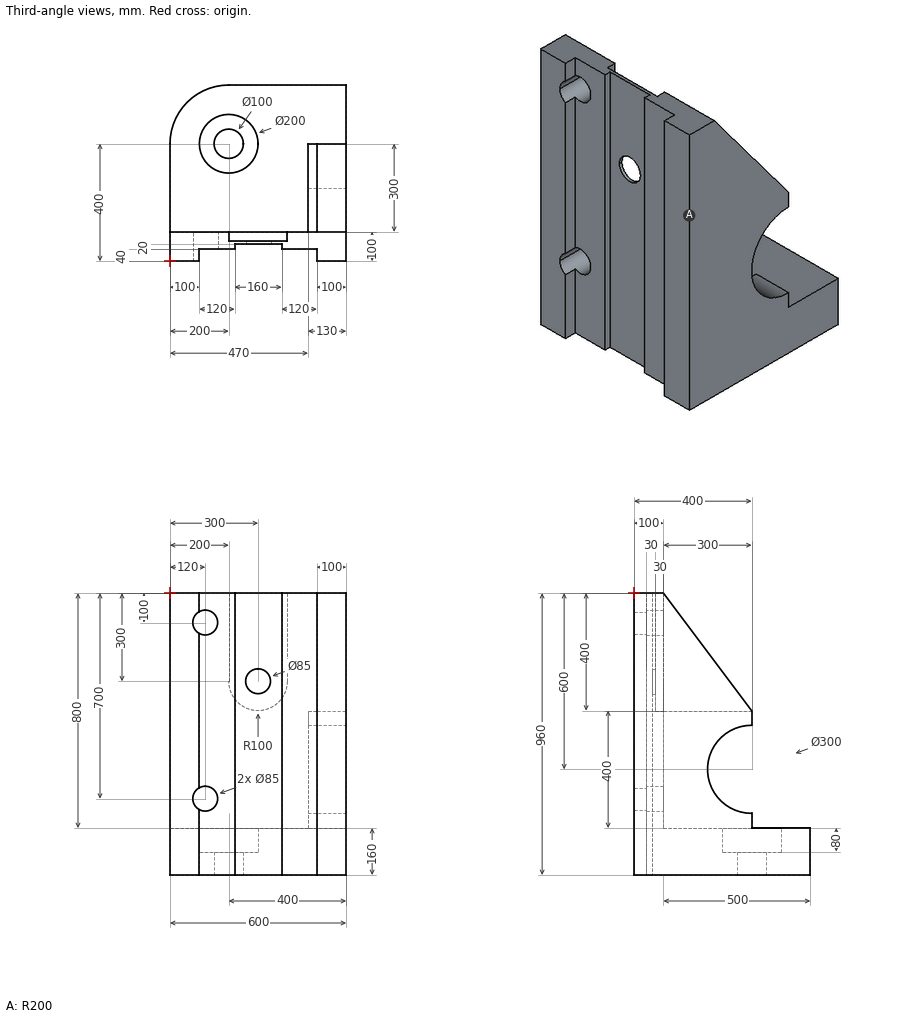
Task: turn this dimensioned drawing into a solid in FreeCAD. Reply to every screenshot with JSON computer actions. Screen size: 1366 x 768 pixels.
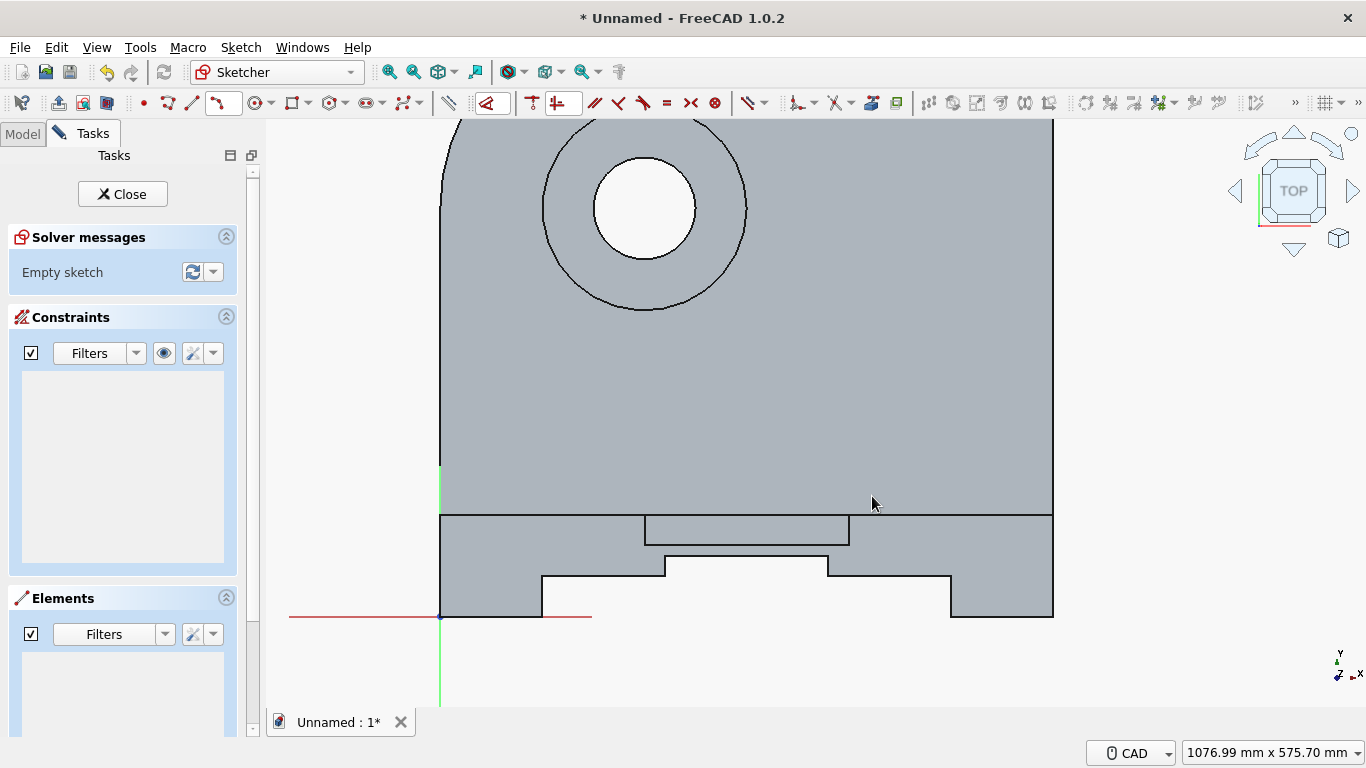
{"action": "left_click", "coordinate": [292, 104]}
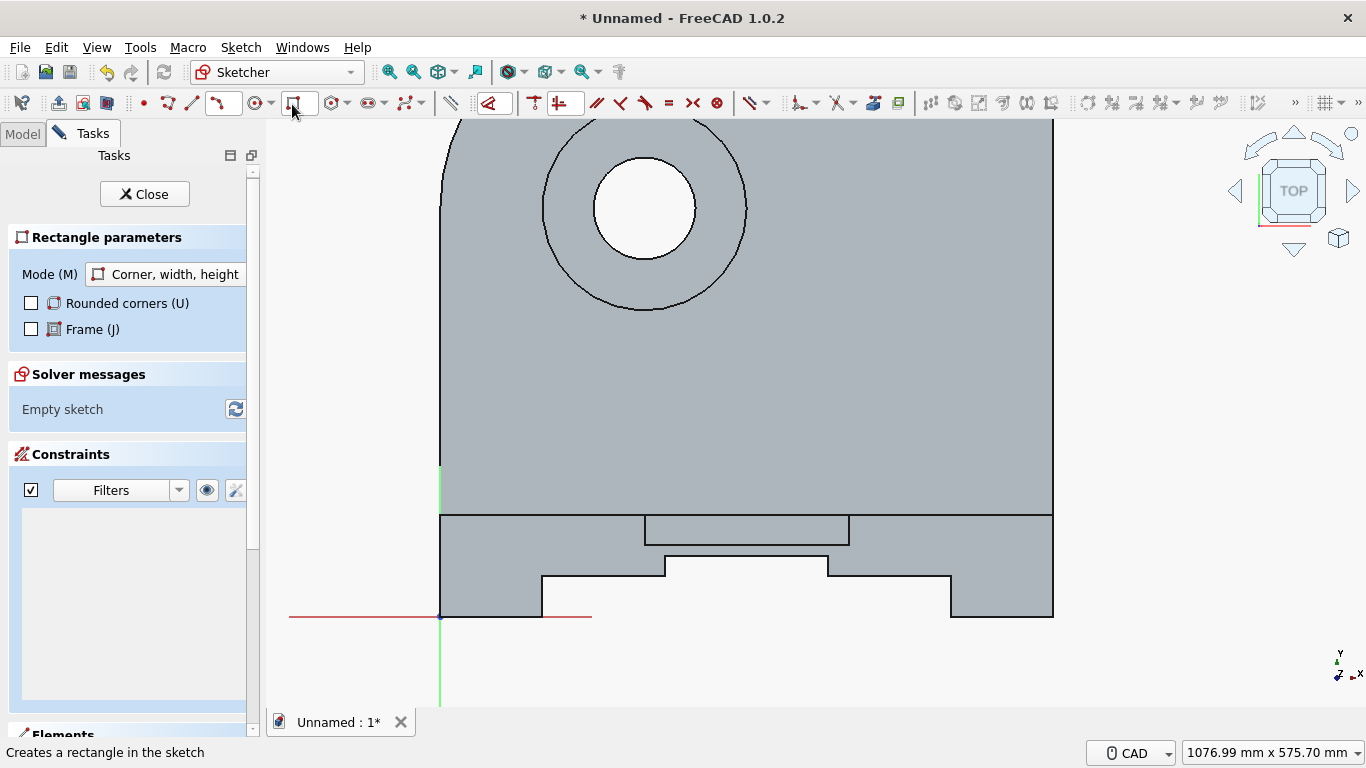
{"action": "left_click", "coordinate": [920, 208]}
{"action": "left_click", "coordinate": [1053, 515]}
{"action": "key", "text": "Escape"}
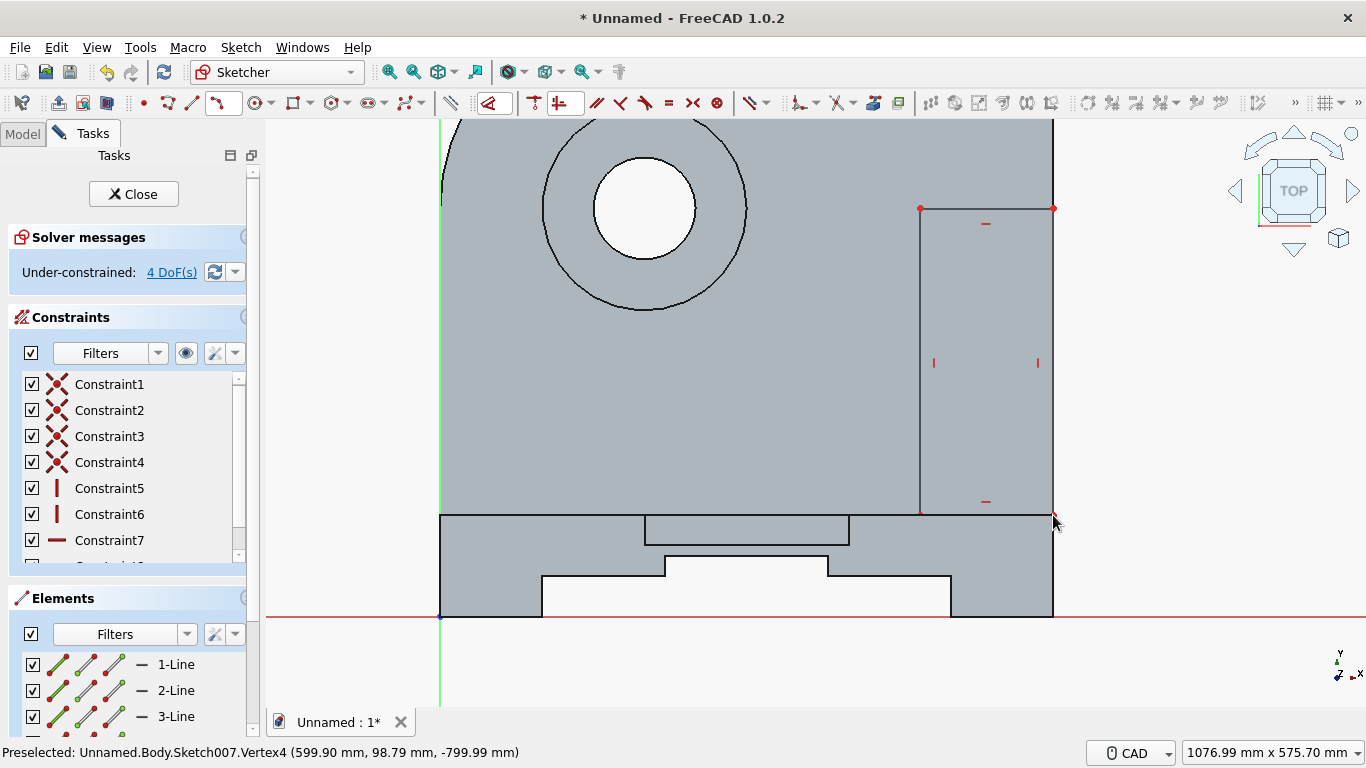
{"action": "left_click", "coordinate": [920, 301]}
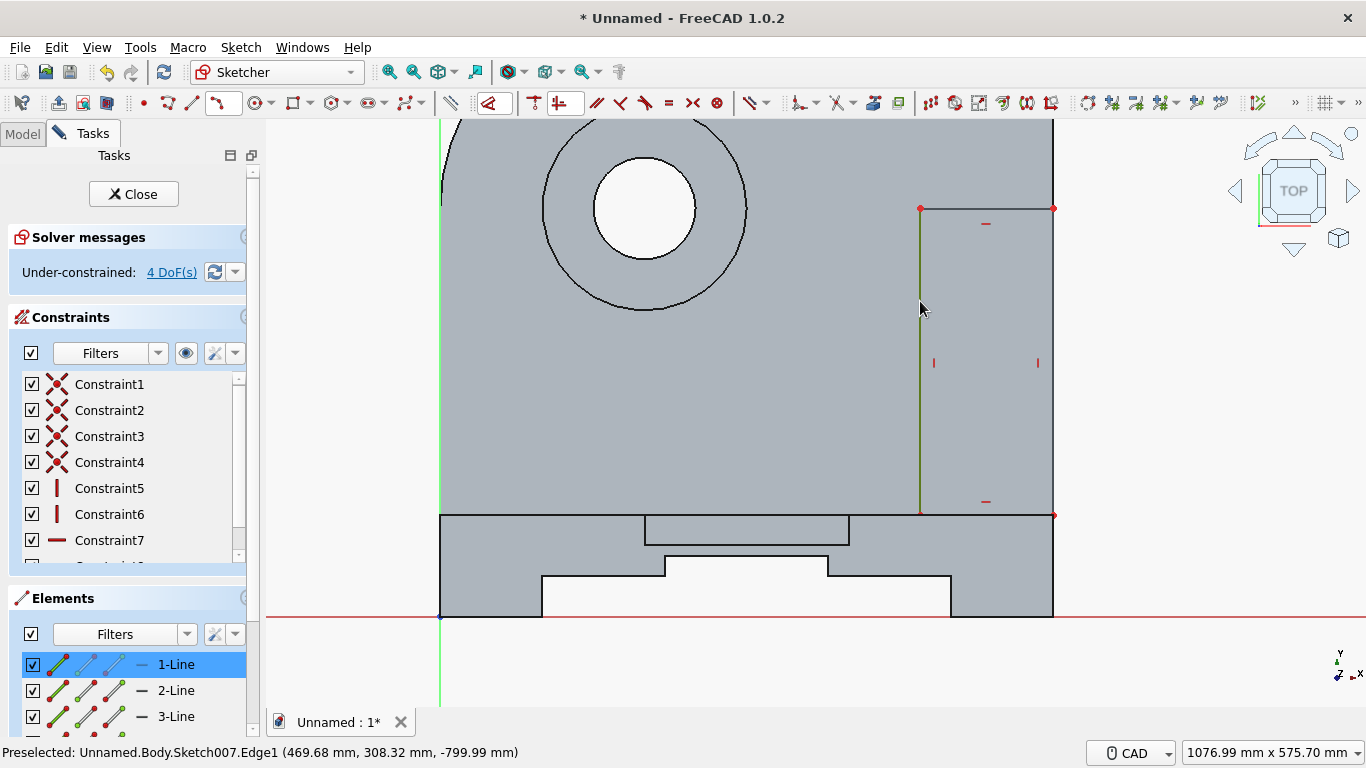
{"action": "left_click", "coordinate": [506, 104]}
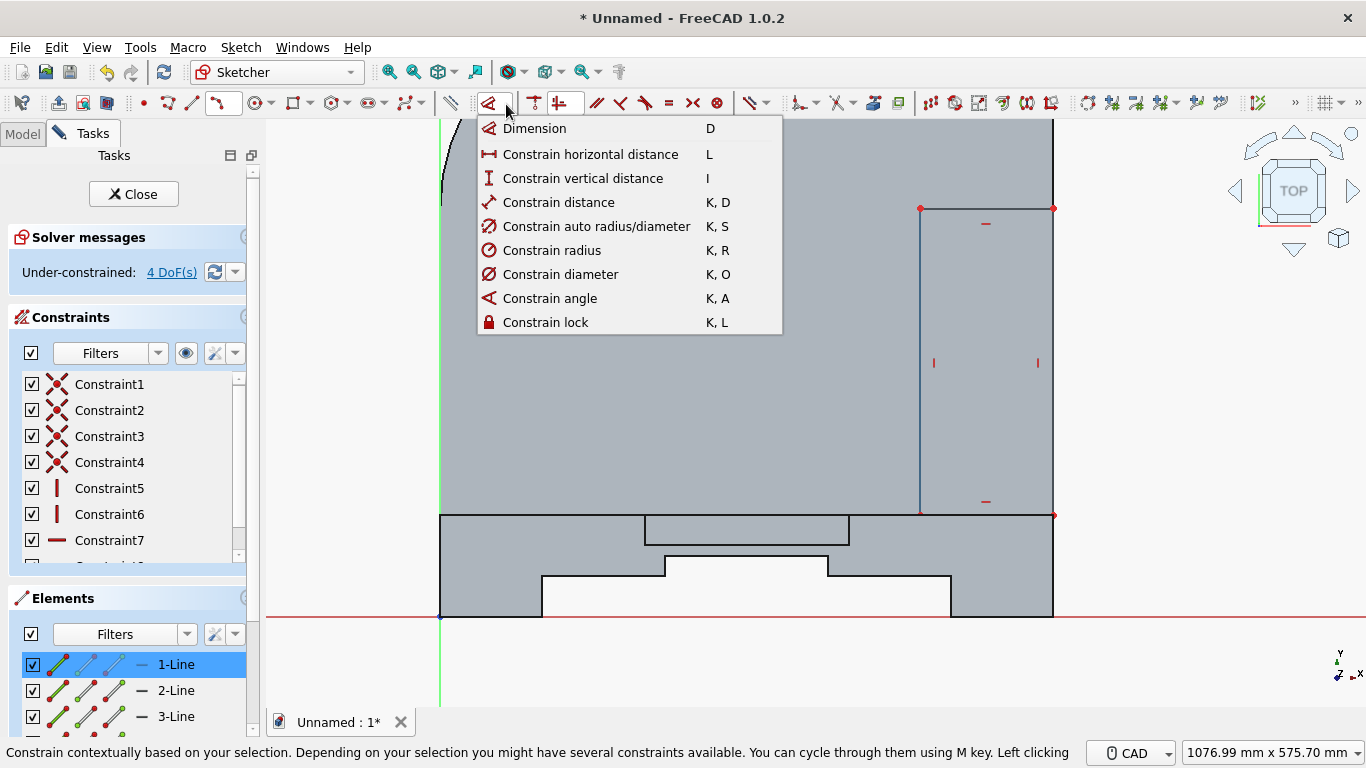
{"action": "left_click", "coordinate": [630, 178]}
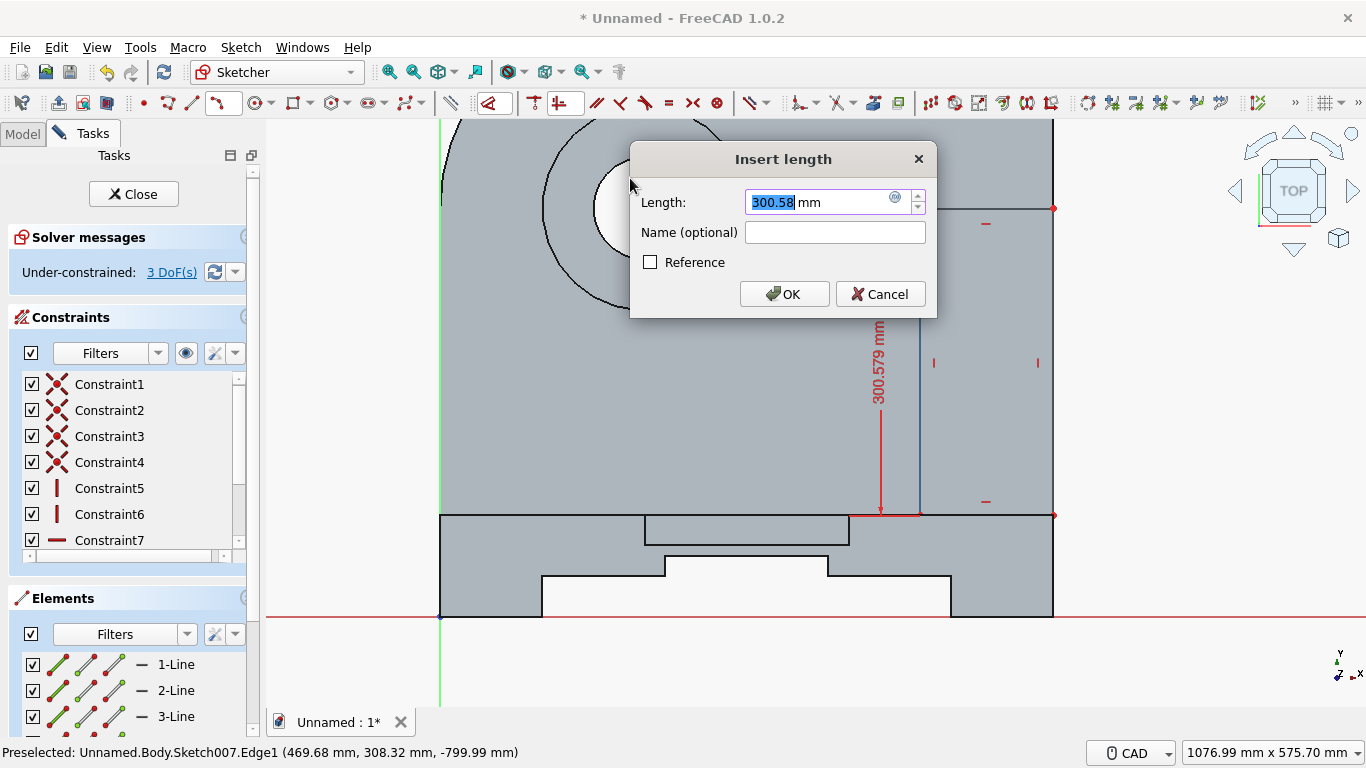
{"action": "type", "text": "300"}
{"action": "key", "text": "Return"}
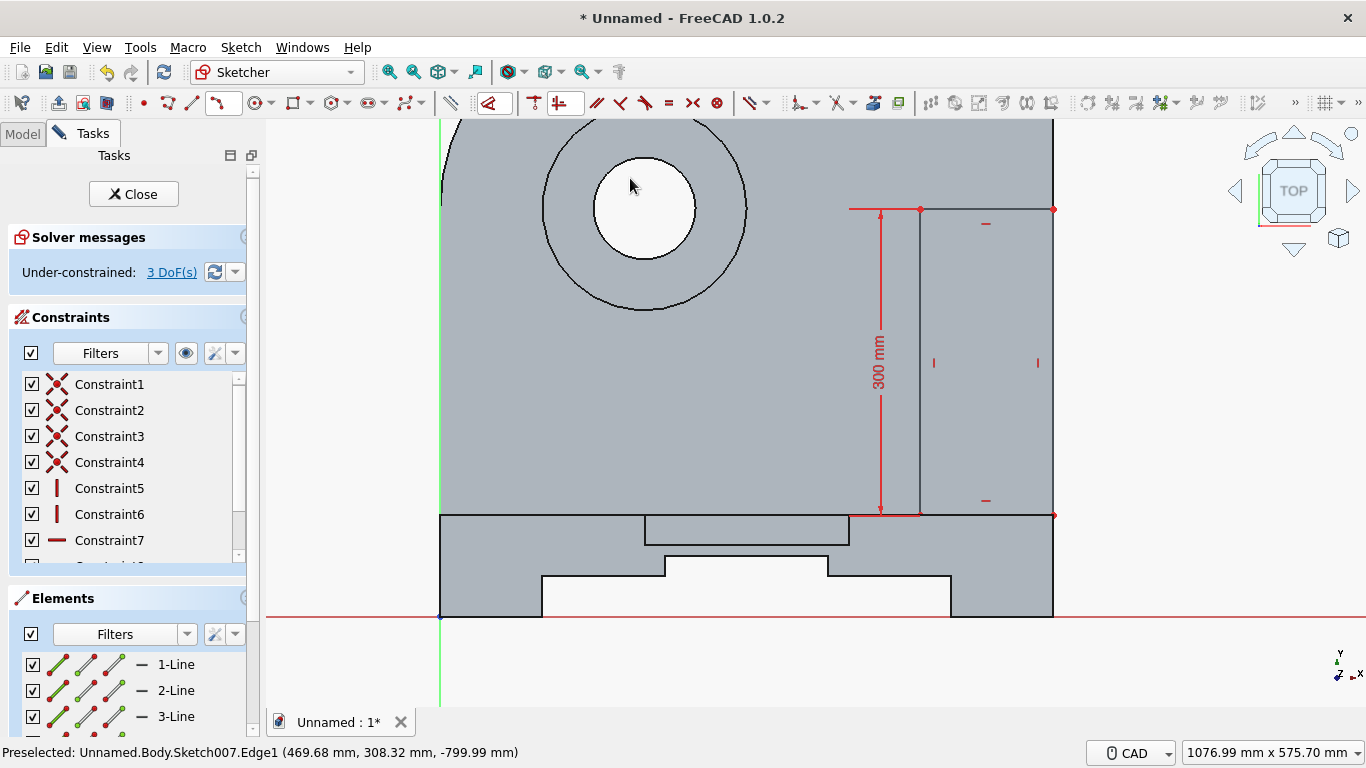
{"action": "left_click", "coordinate": [960, 516]}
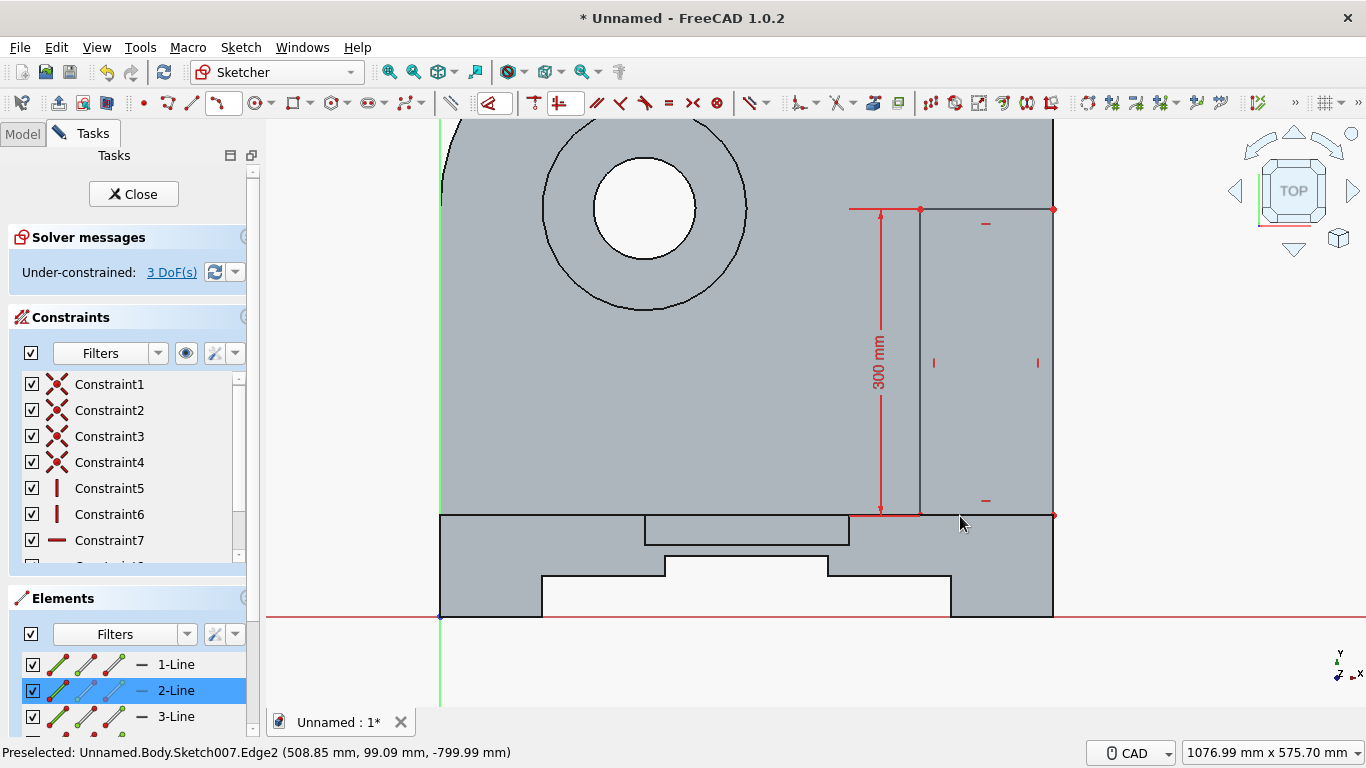
{"action": "key", "text": "l"}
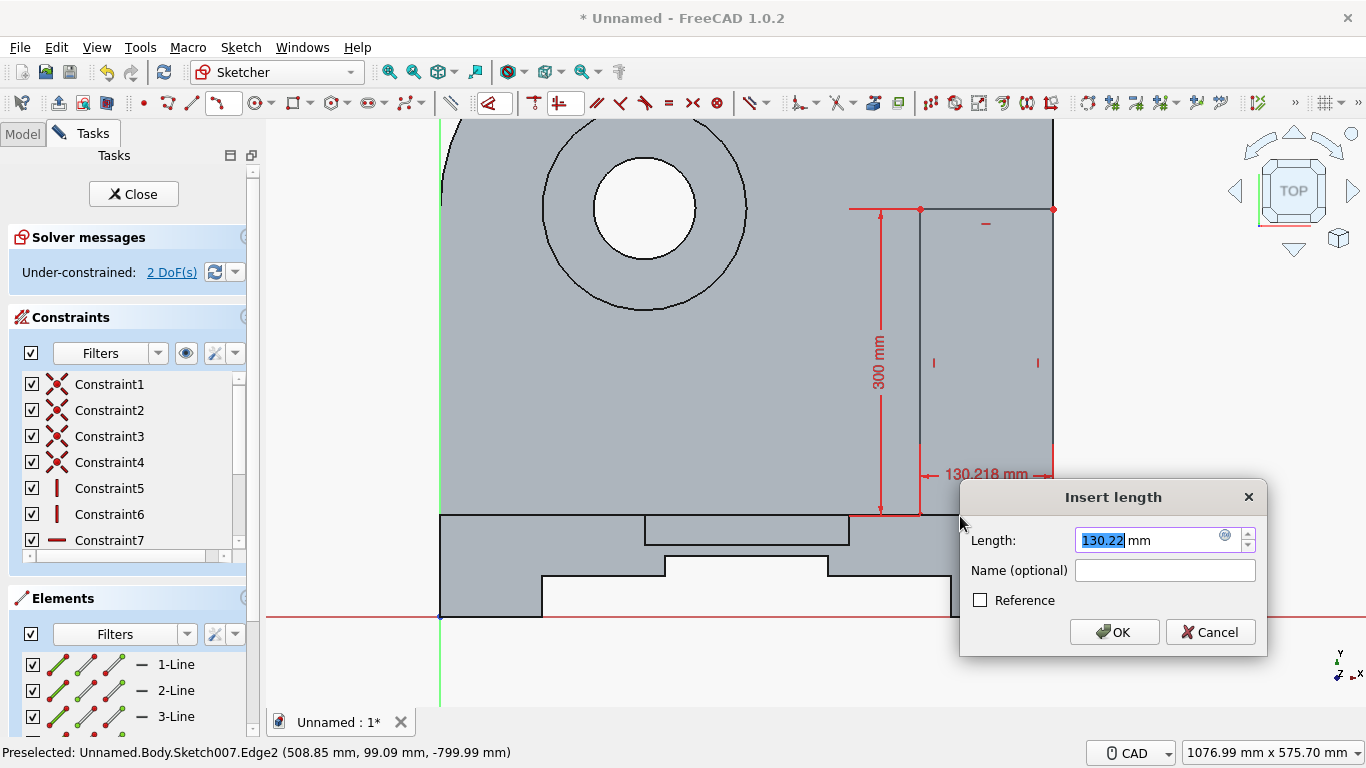
{"action": "type", "text": "130"}
{"action": "key", "text": "Return"}